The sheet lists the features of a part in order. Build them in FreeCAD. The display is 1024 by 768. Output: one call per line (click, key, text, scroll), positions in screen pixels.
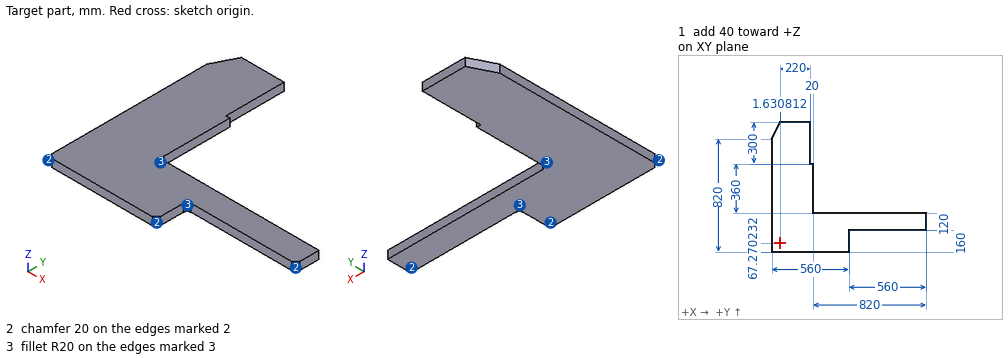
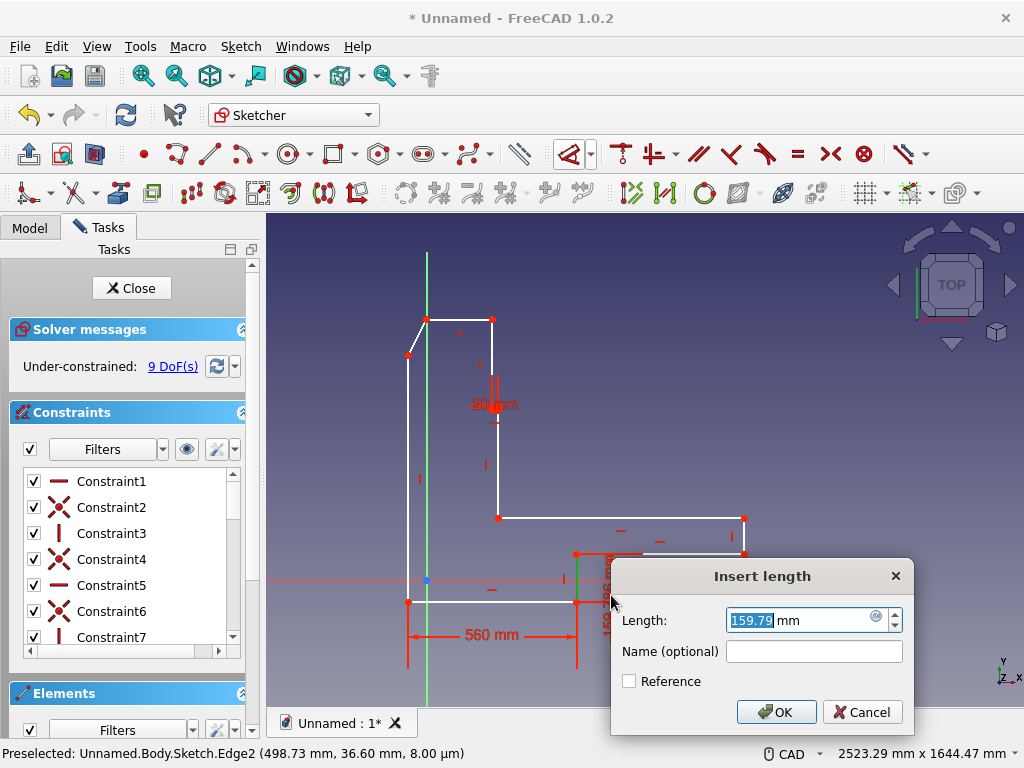
text(160)
key(Return)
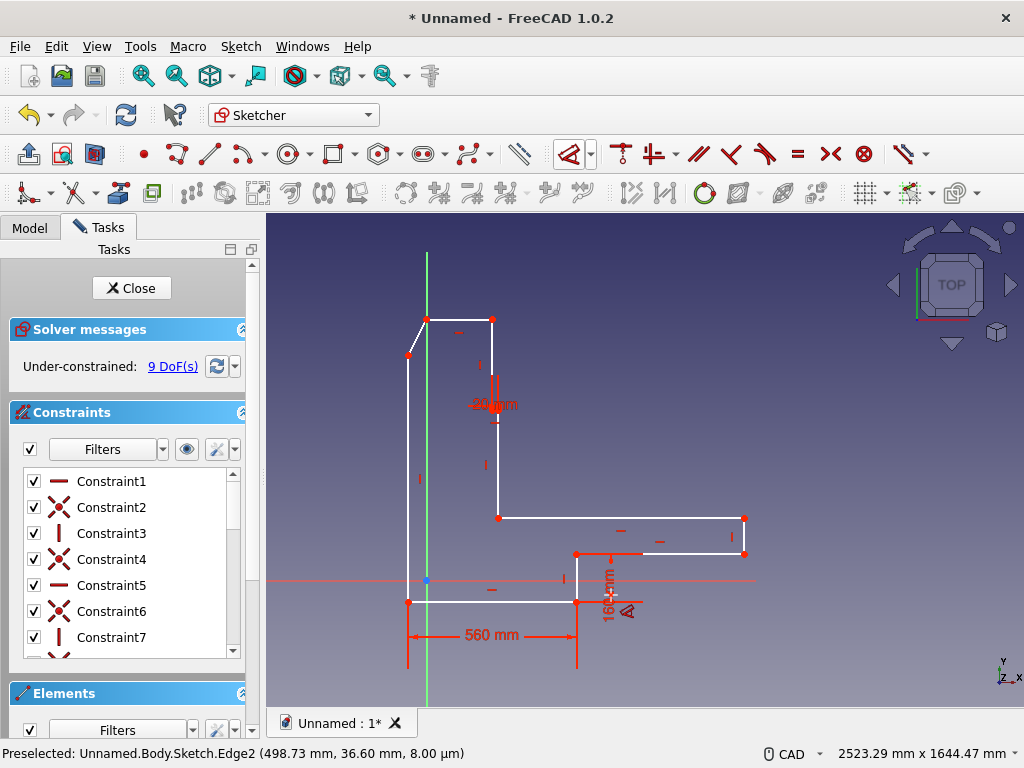
click(627, 554)
click(699, 612)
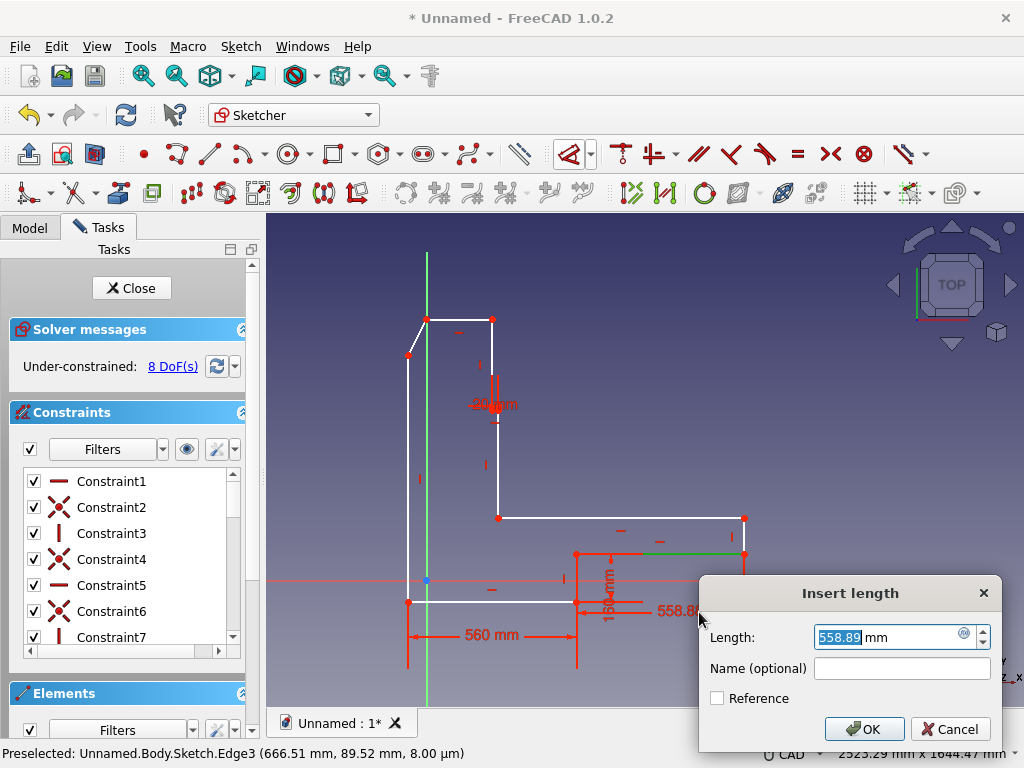
text(560)
key(Return)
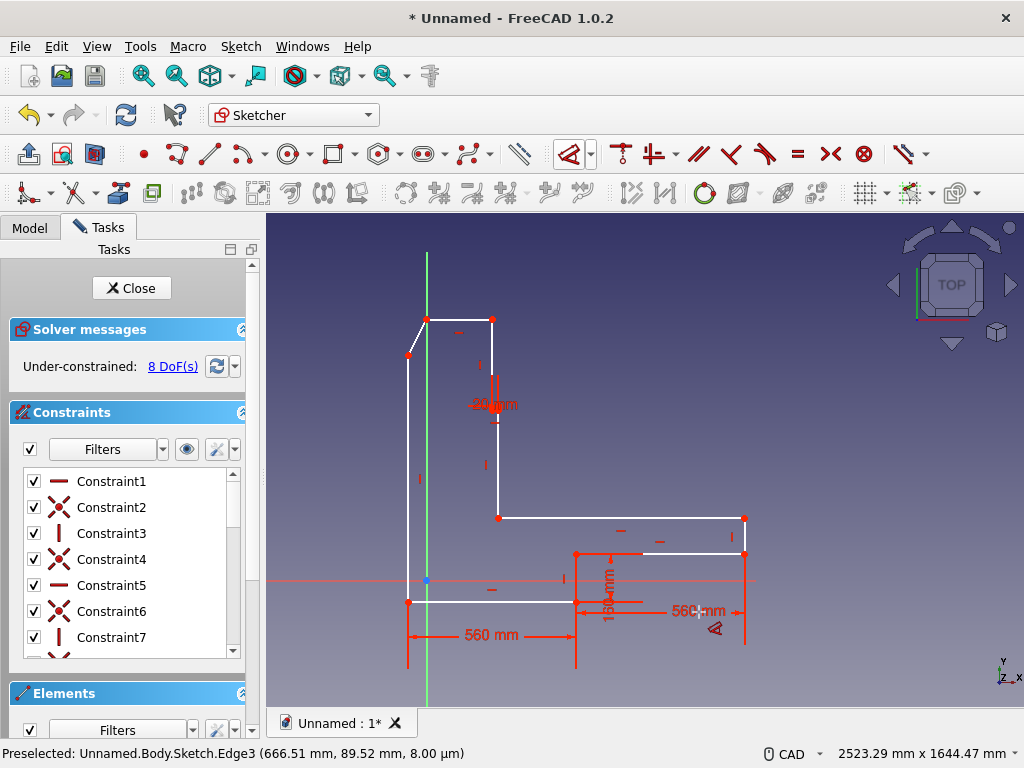
scroll(745, 543, up, 2)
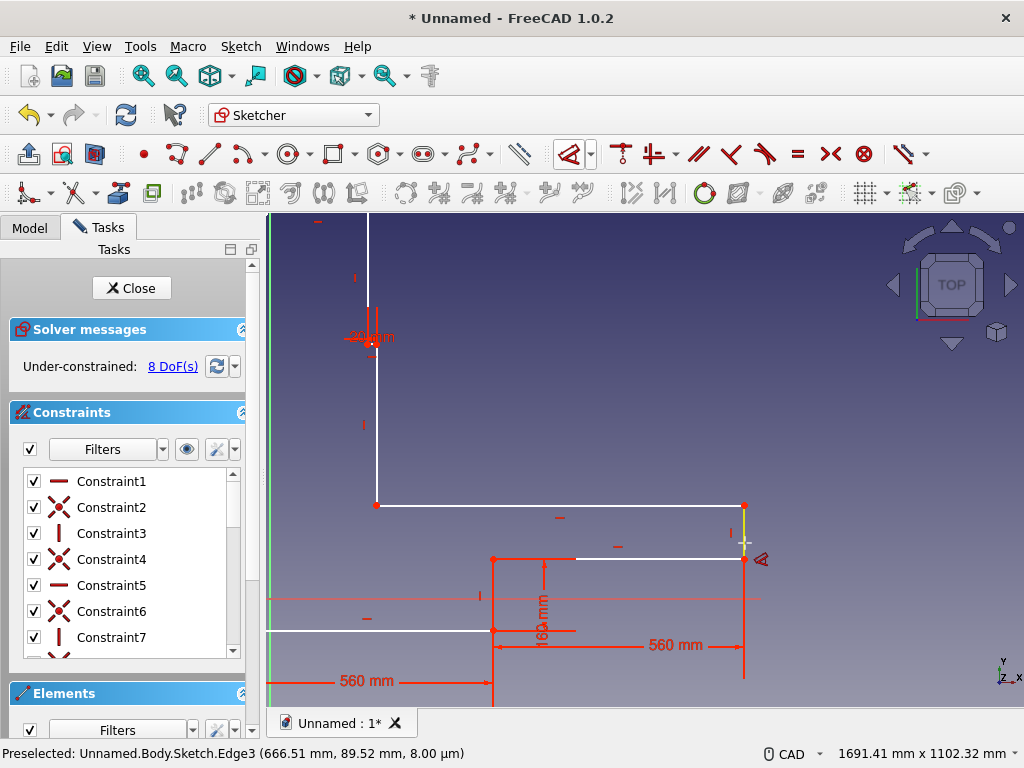
click(744, 543)
click(778, 532)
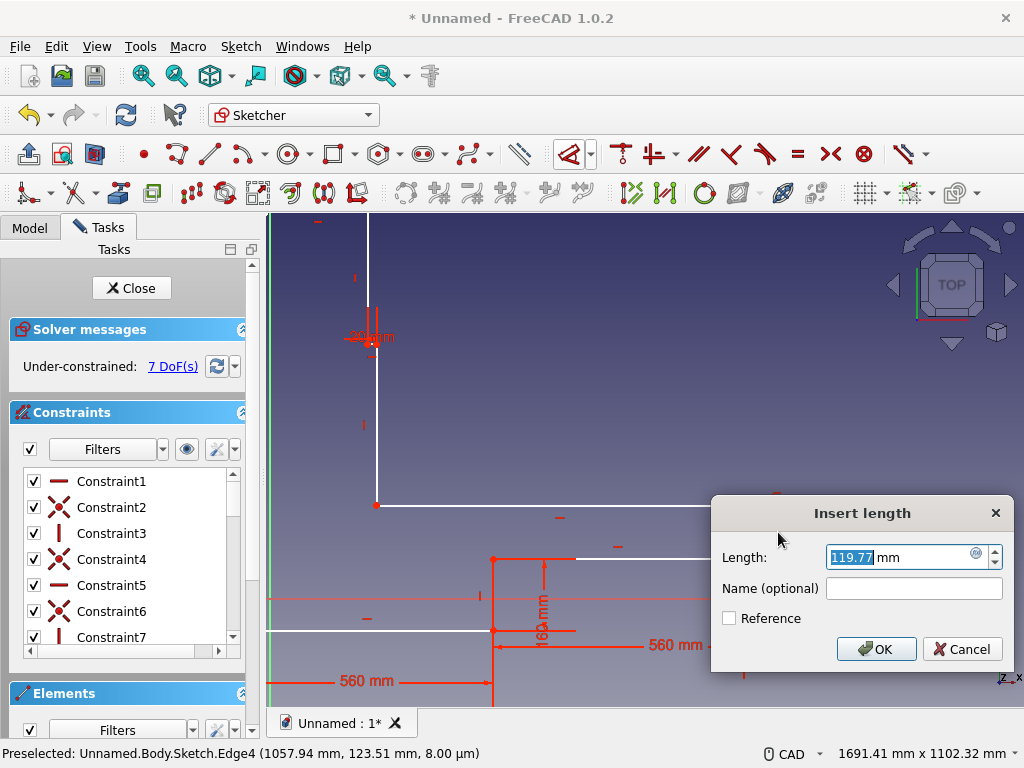
text(120)
key(Return)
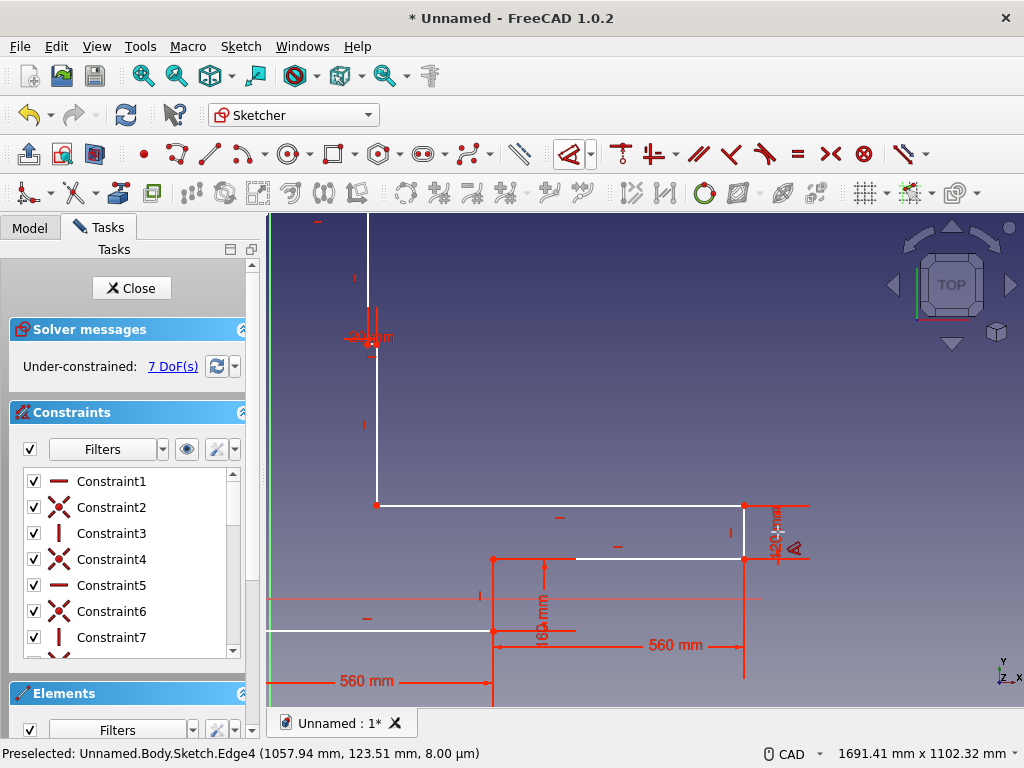
click(634, 506)
click(560, 540)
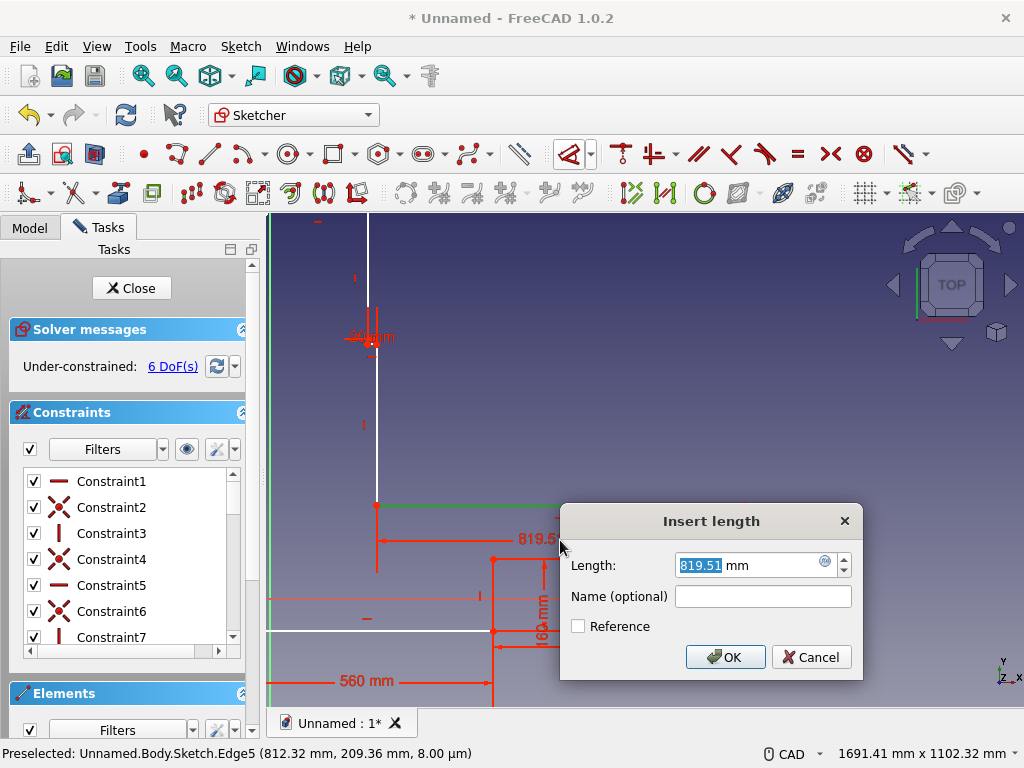
text(820)
key(Return)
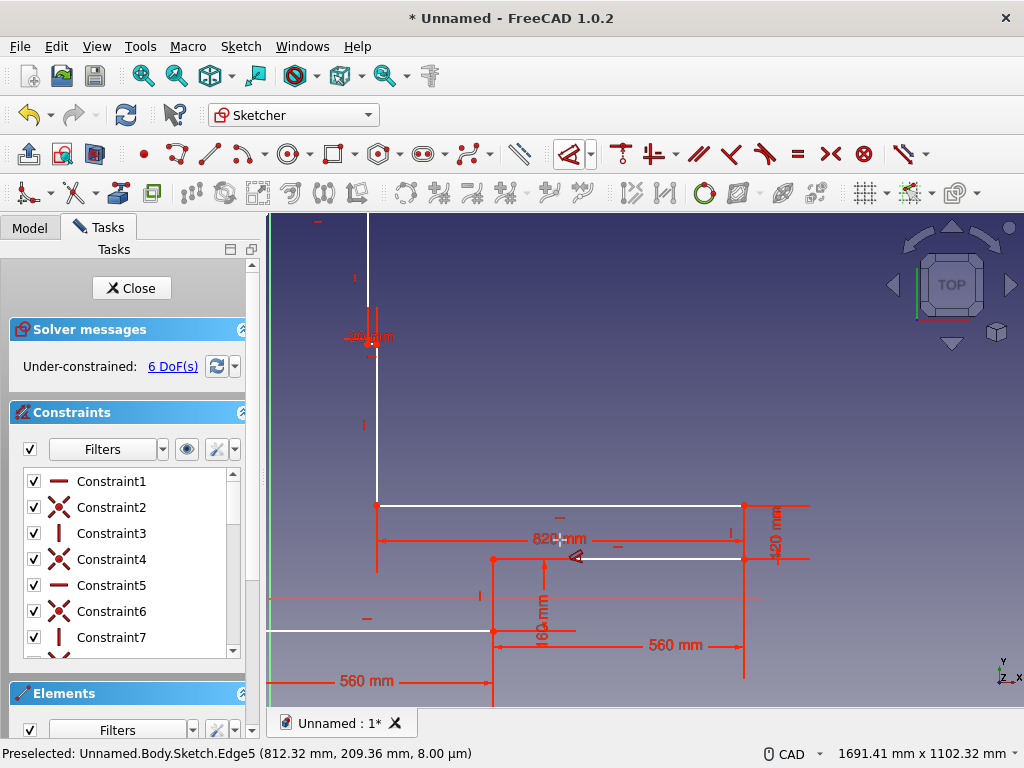
click(377, 457)
click(343, 425)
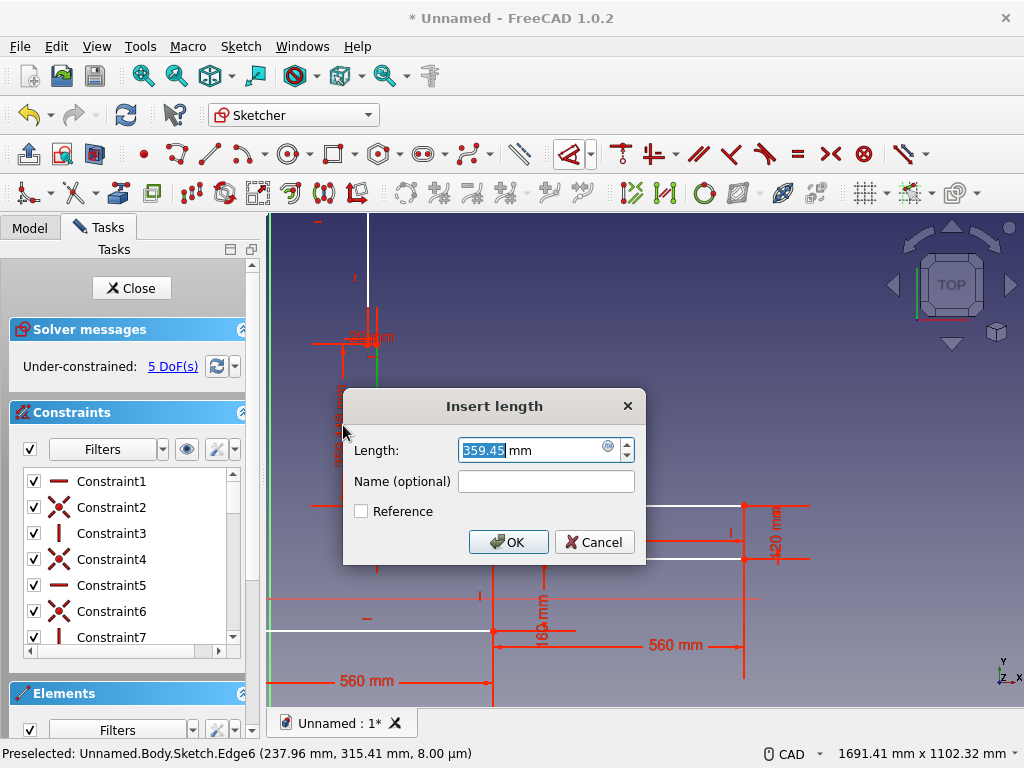
text(360)
key(Return)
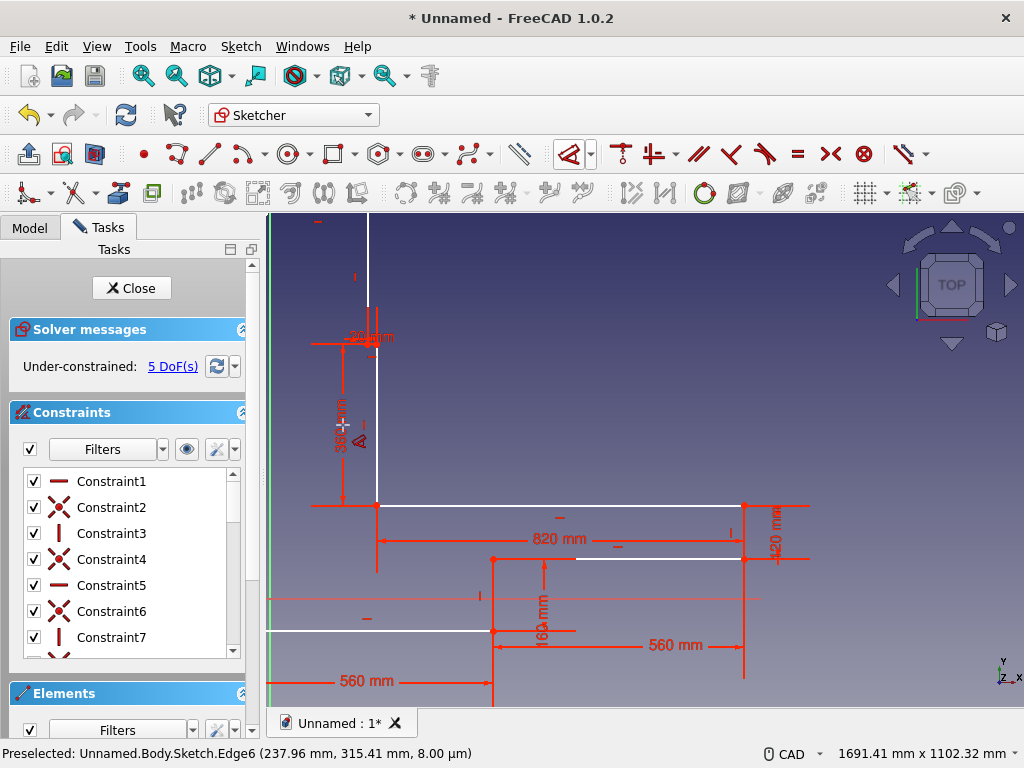
click(368, 304)
click(334, 293)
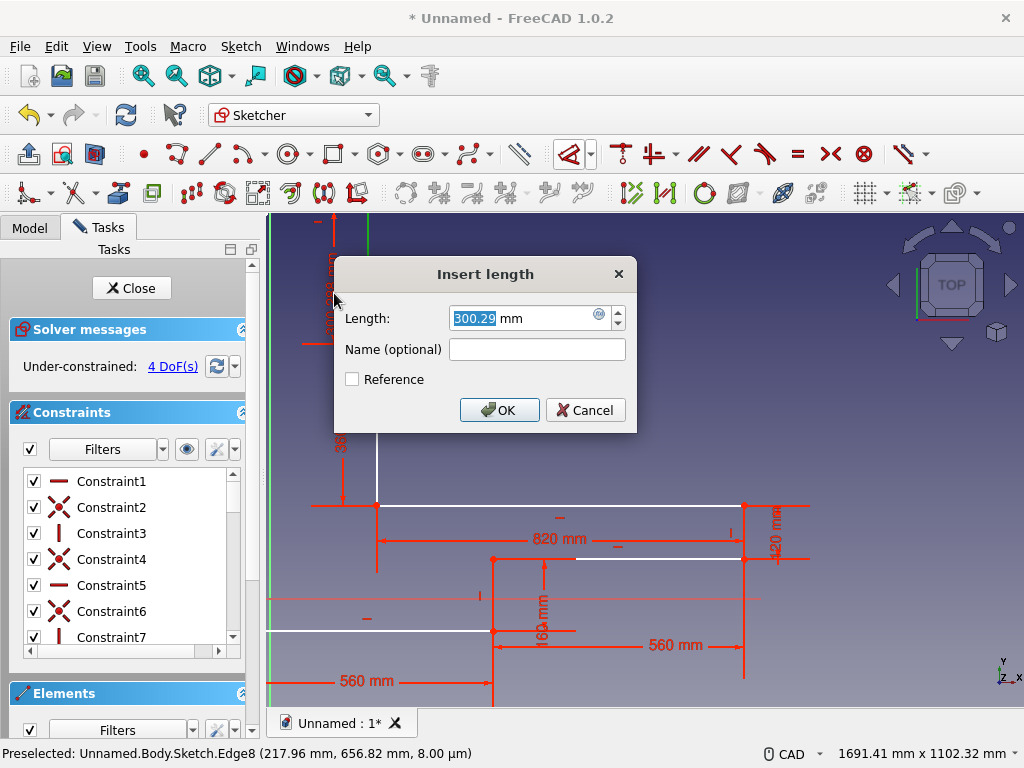
text(300)
key(Return)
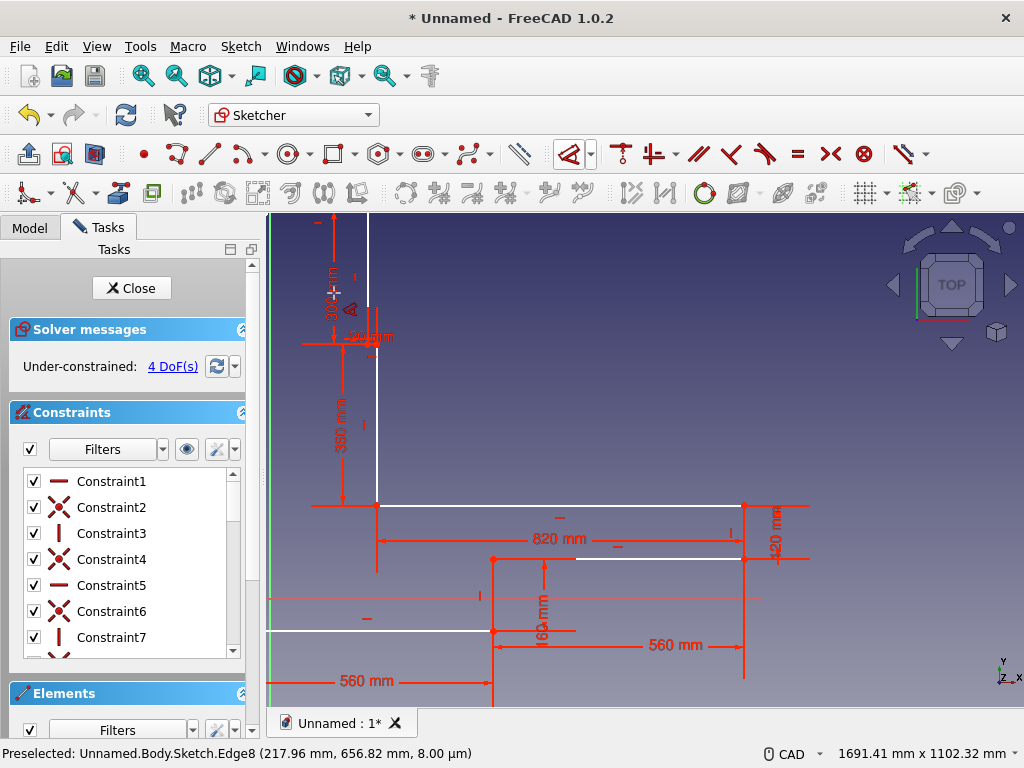
scroll(746, 544, down, 2)